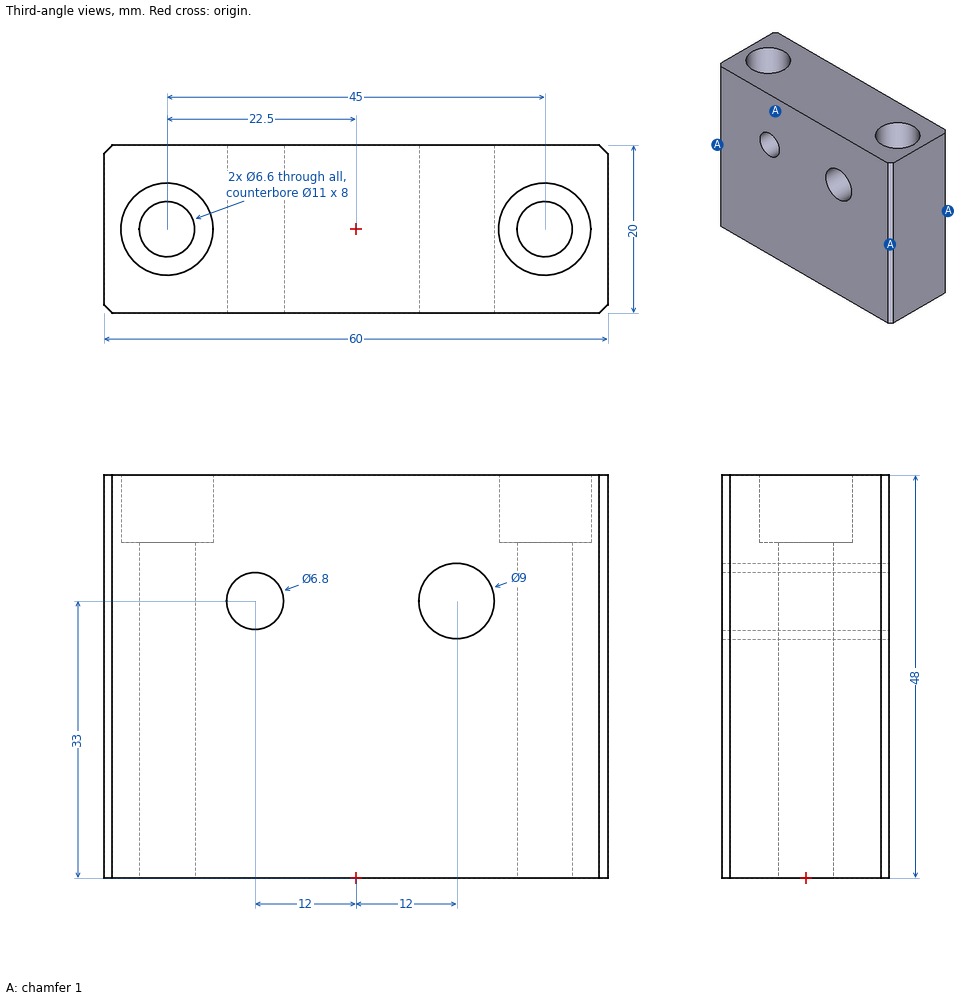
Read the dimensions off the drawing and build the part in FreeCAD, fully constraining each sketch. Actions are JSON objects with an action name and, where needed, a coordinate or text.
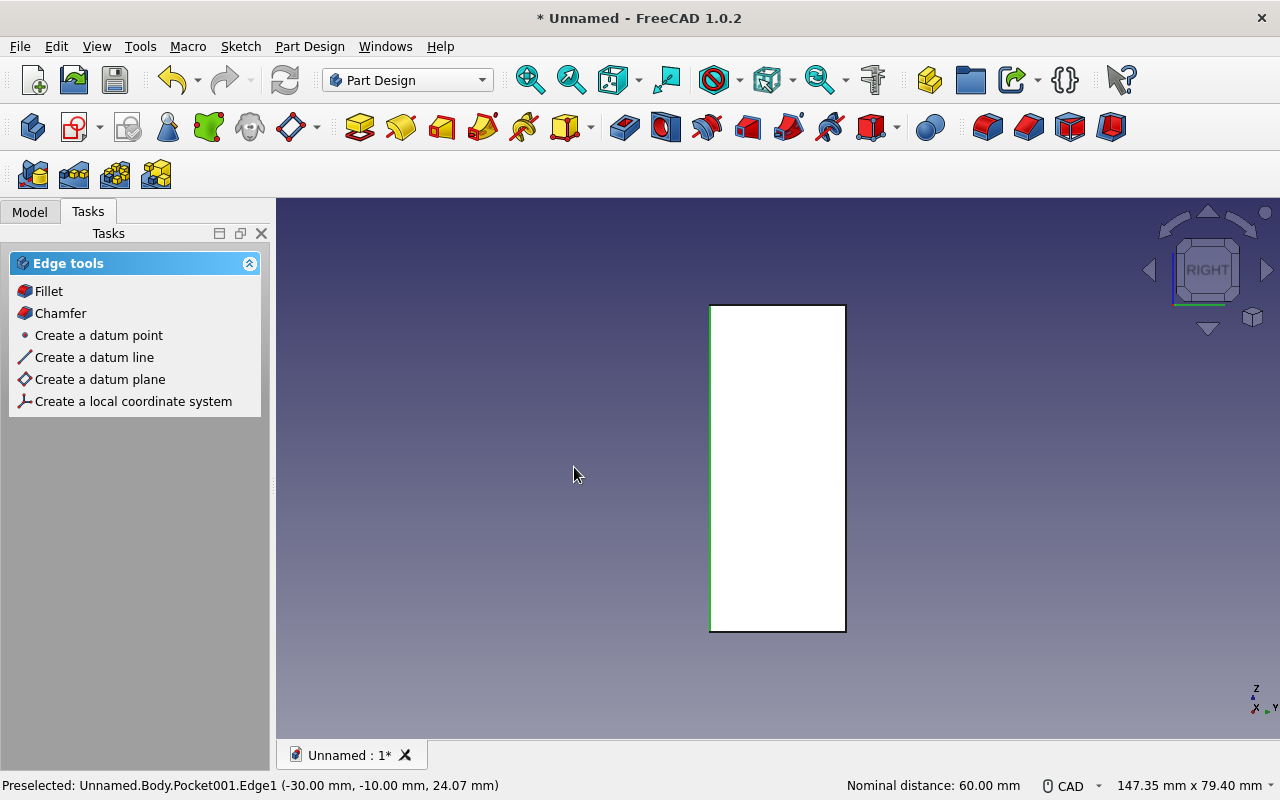
{"action": "left_click", "coordinate": [846, 467], "text": "ctrl"}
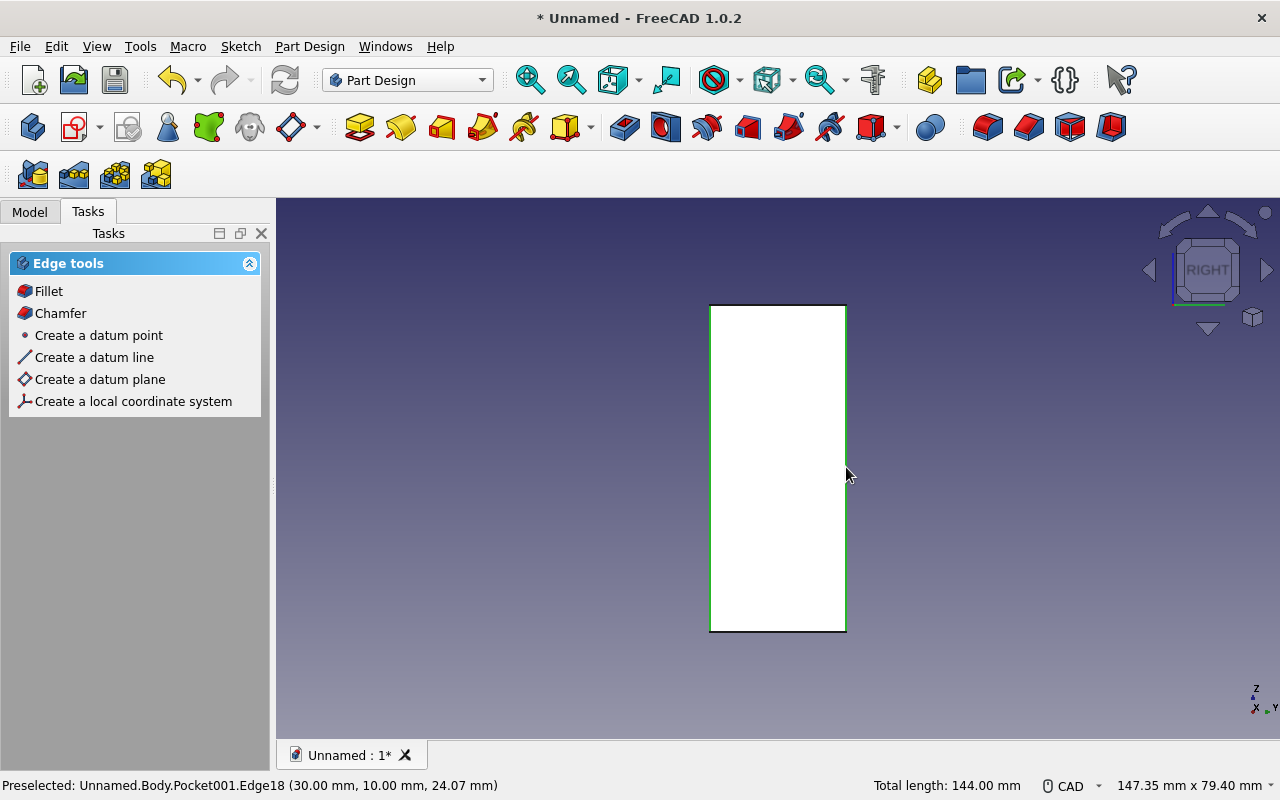
{"action": "key", "text": "5"}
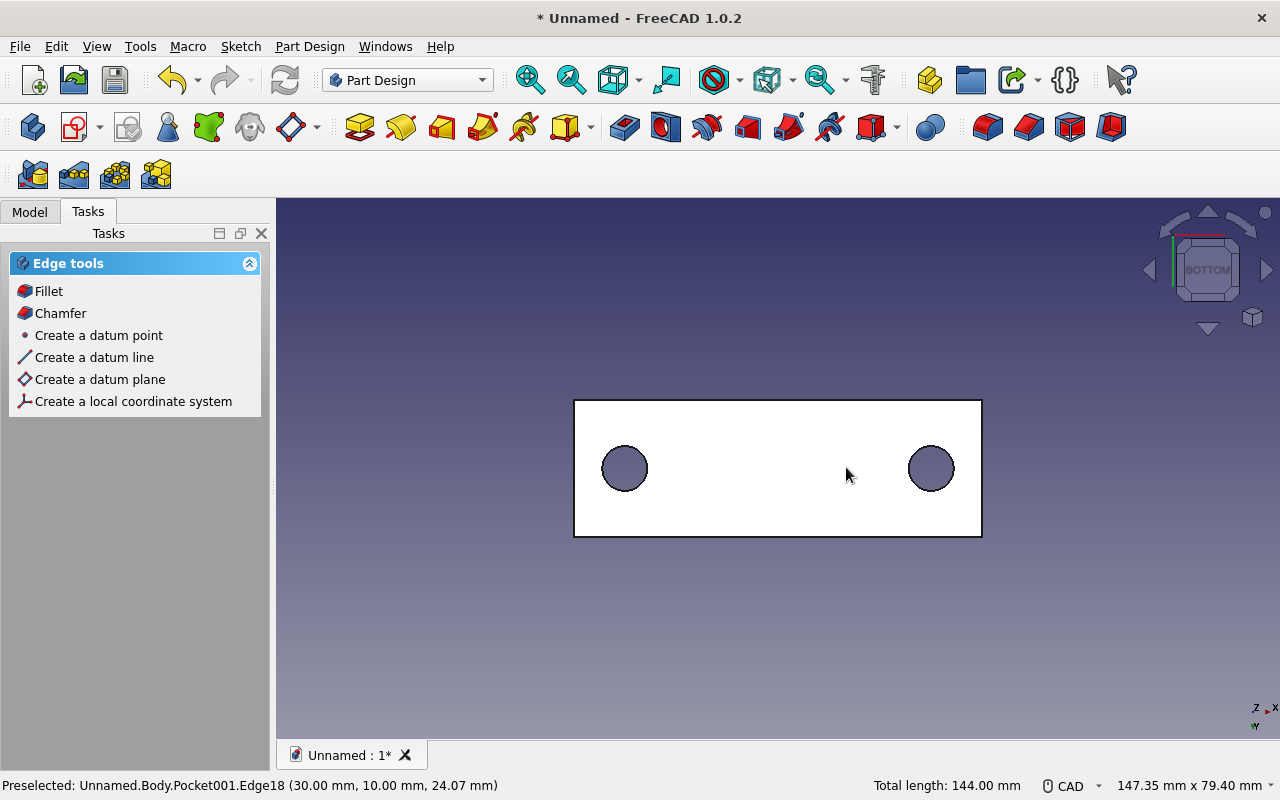
{"action": "left_click", "coordinate": [531, 80]}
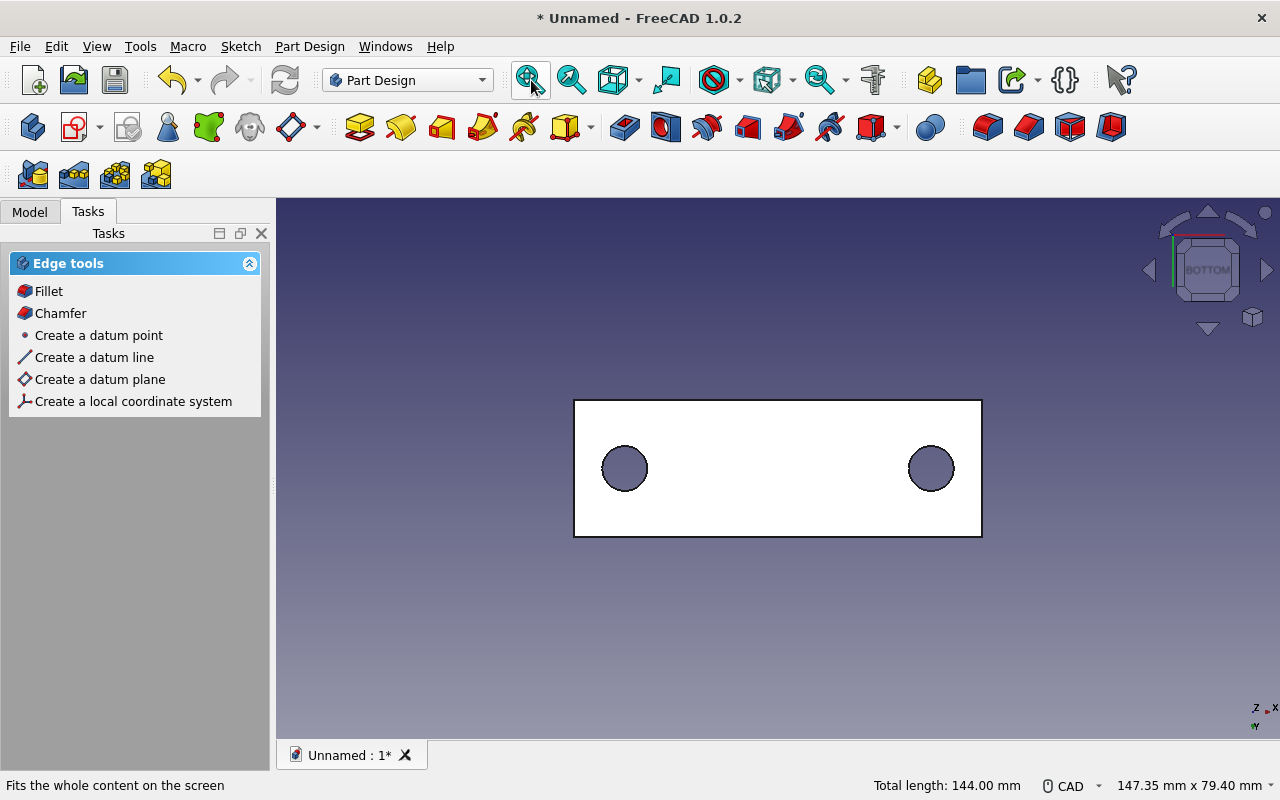
{"action": "key", "text": "4"}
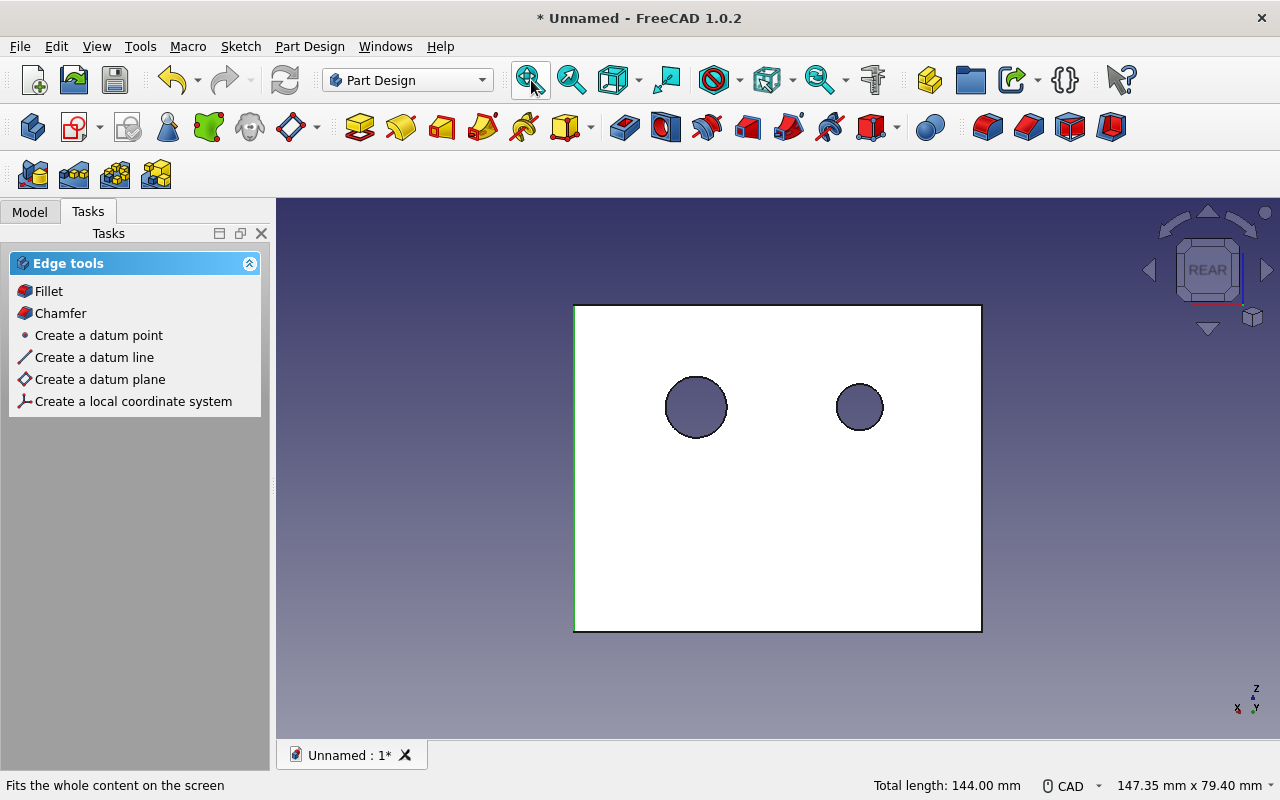
{"action": "left_click", "coordinate": [982, 467], "text": "ctrl"}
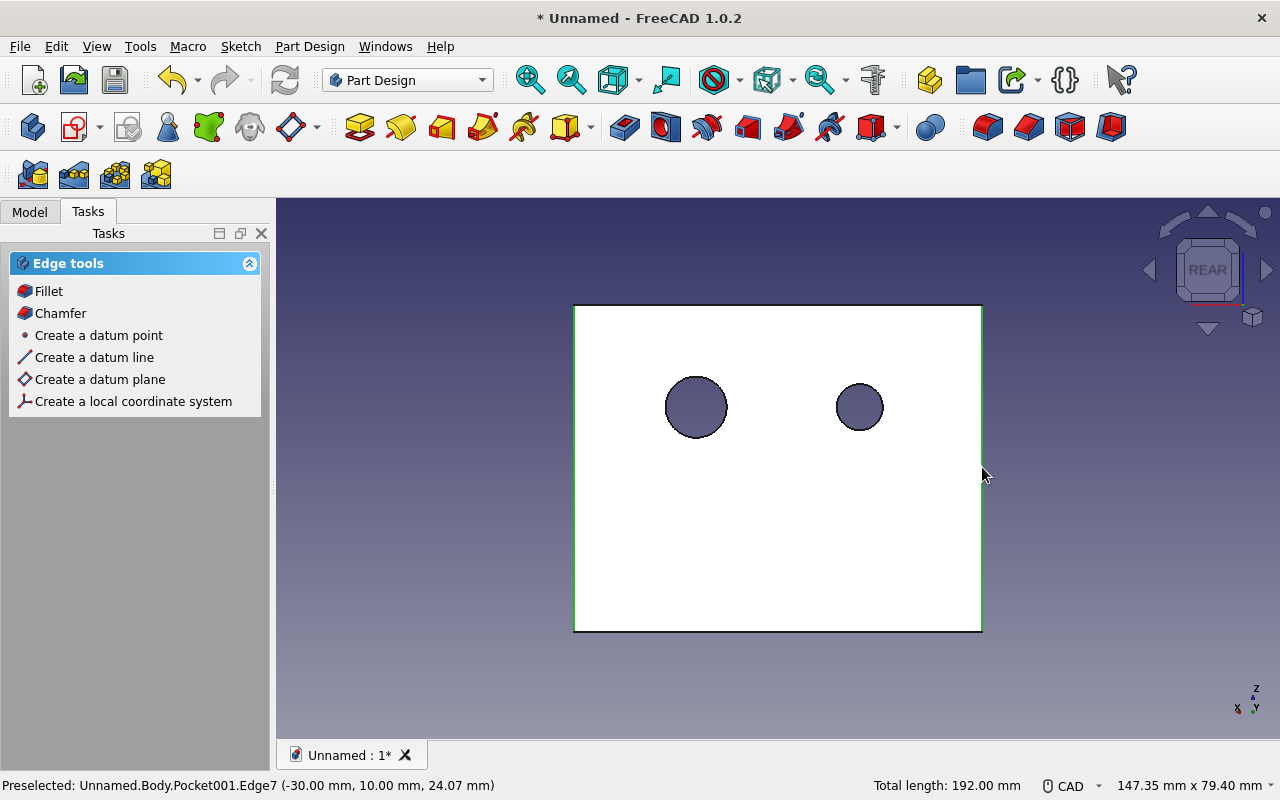
{"action": "left_click", "coordinate": [1029, 128]}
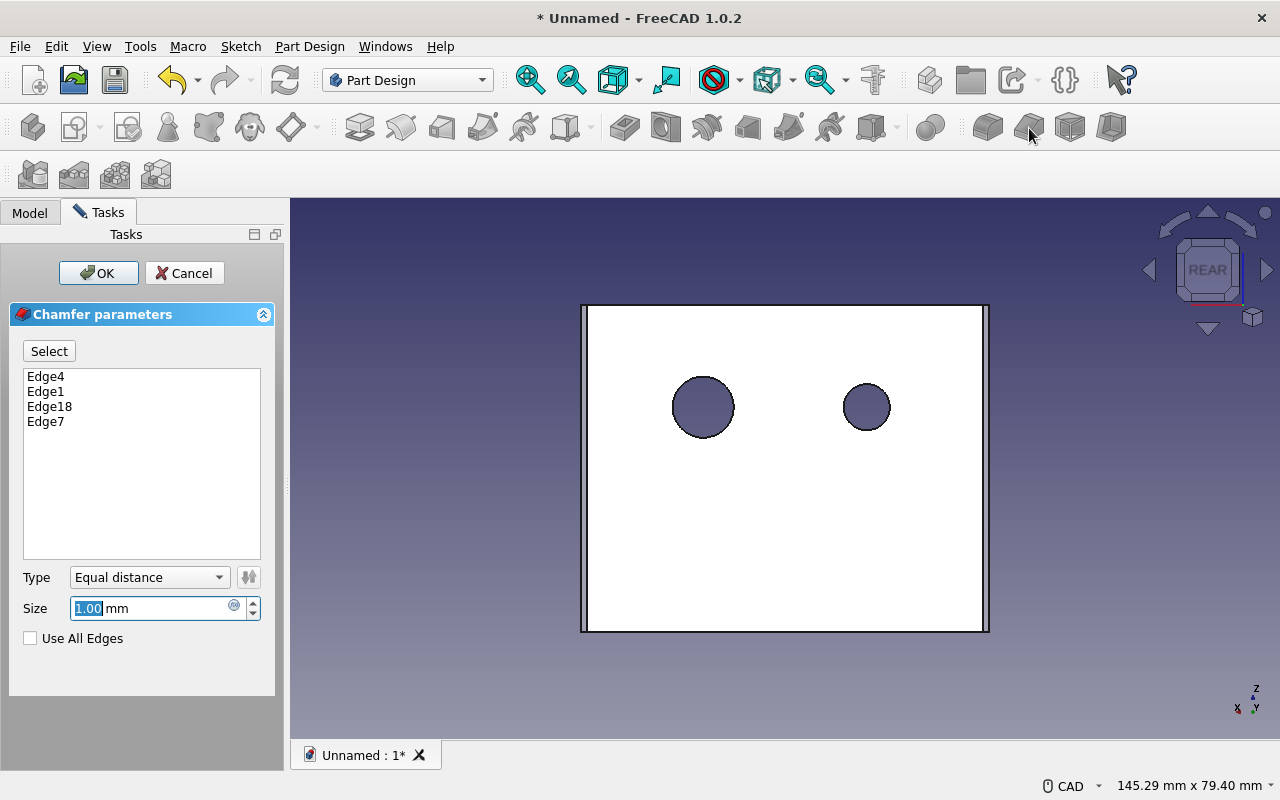
{"action": "type", "text": "1"}
{"action": "key", "text": "Tab"}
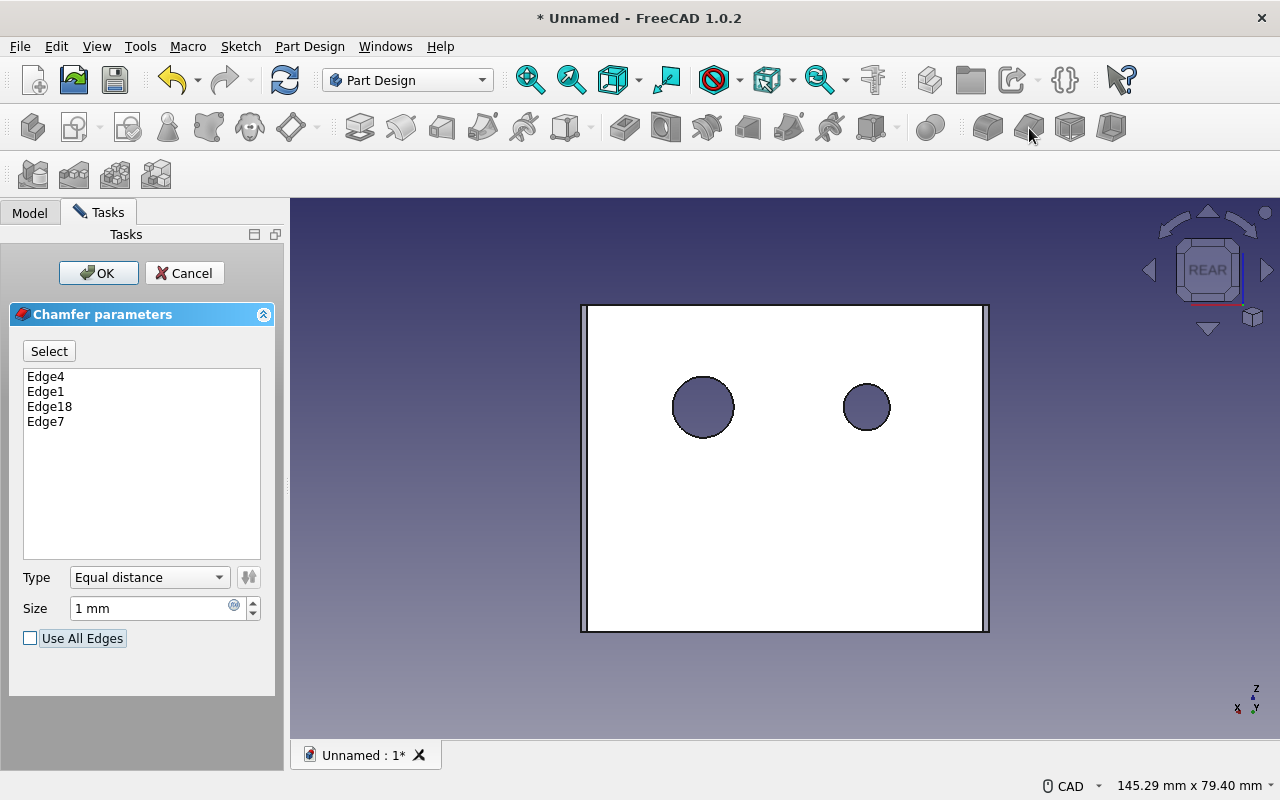
{"action": "left_click", "coordinate": [99, 273]}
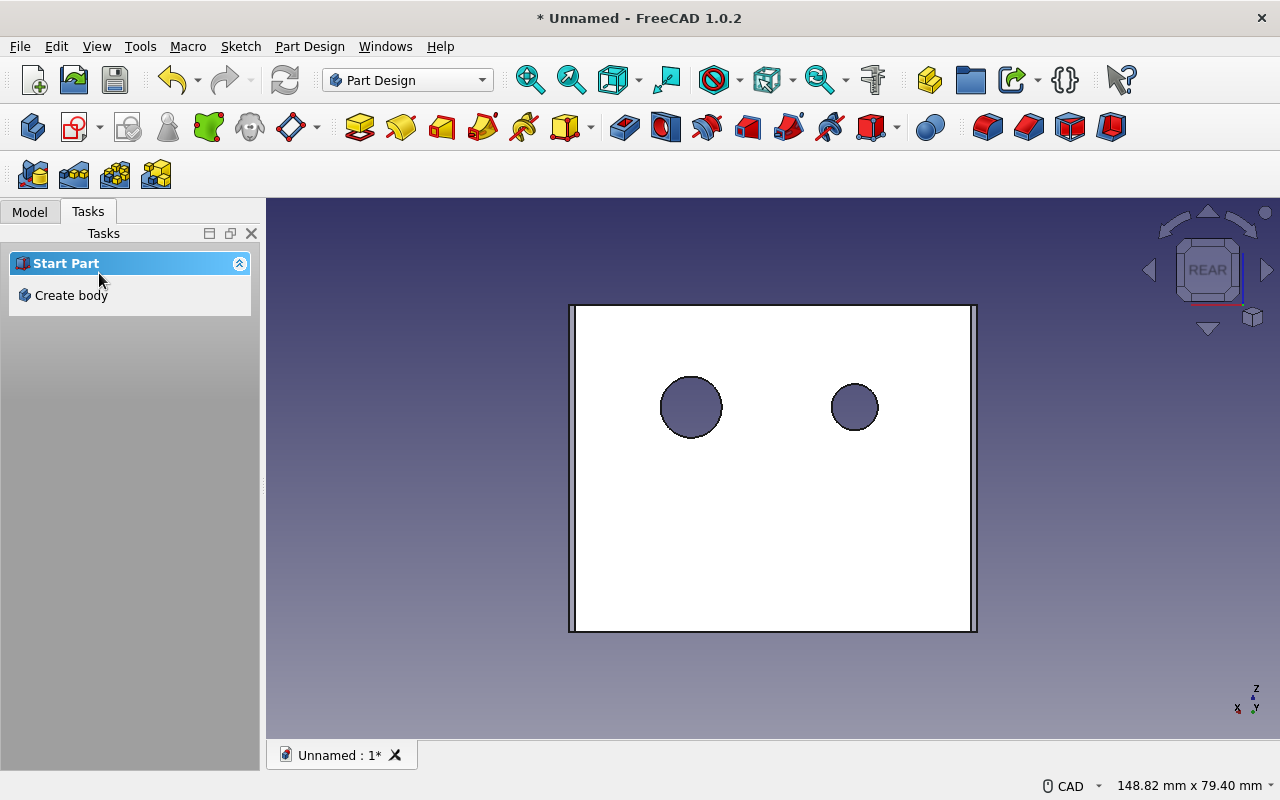
{"action": "key", "text": "0"}